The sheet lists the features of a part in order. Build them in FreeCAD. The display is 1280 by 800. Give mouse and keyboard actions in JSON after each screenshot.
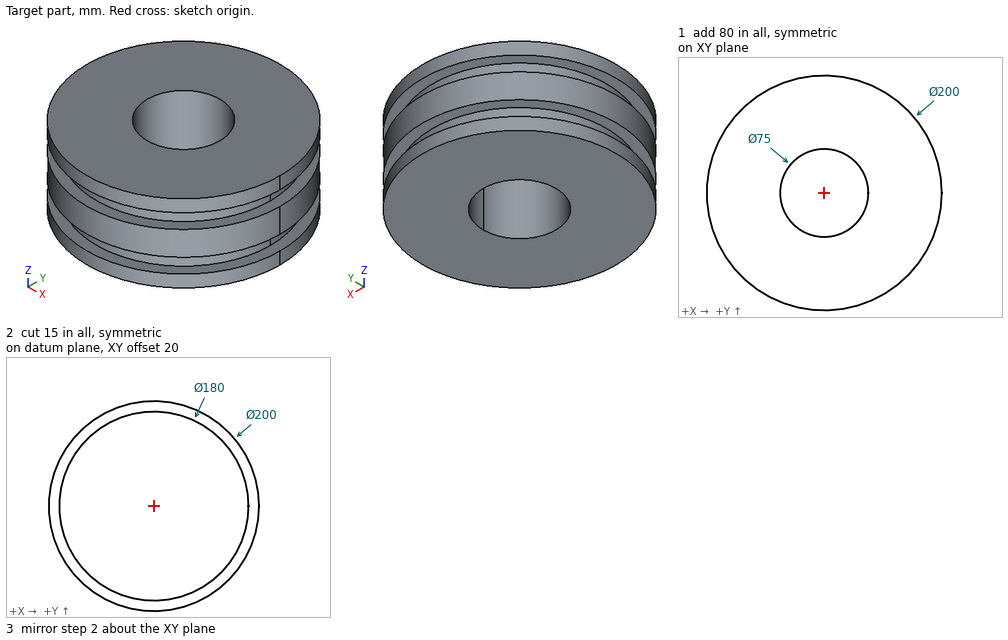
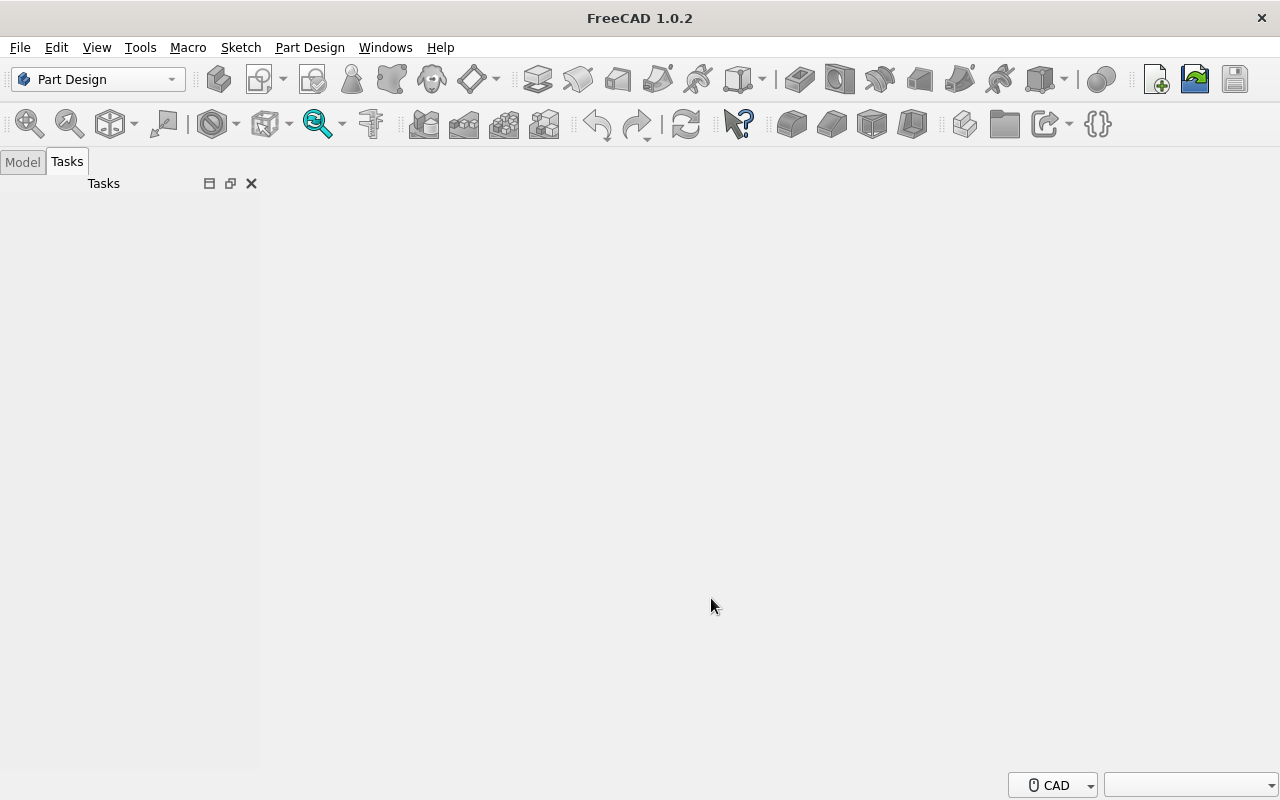
{"action": "left_click", "coordinate": [1156, 80]}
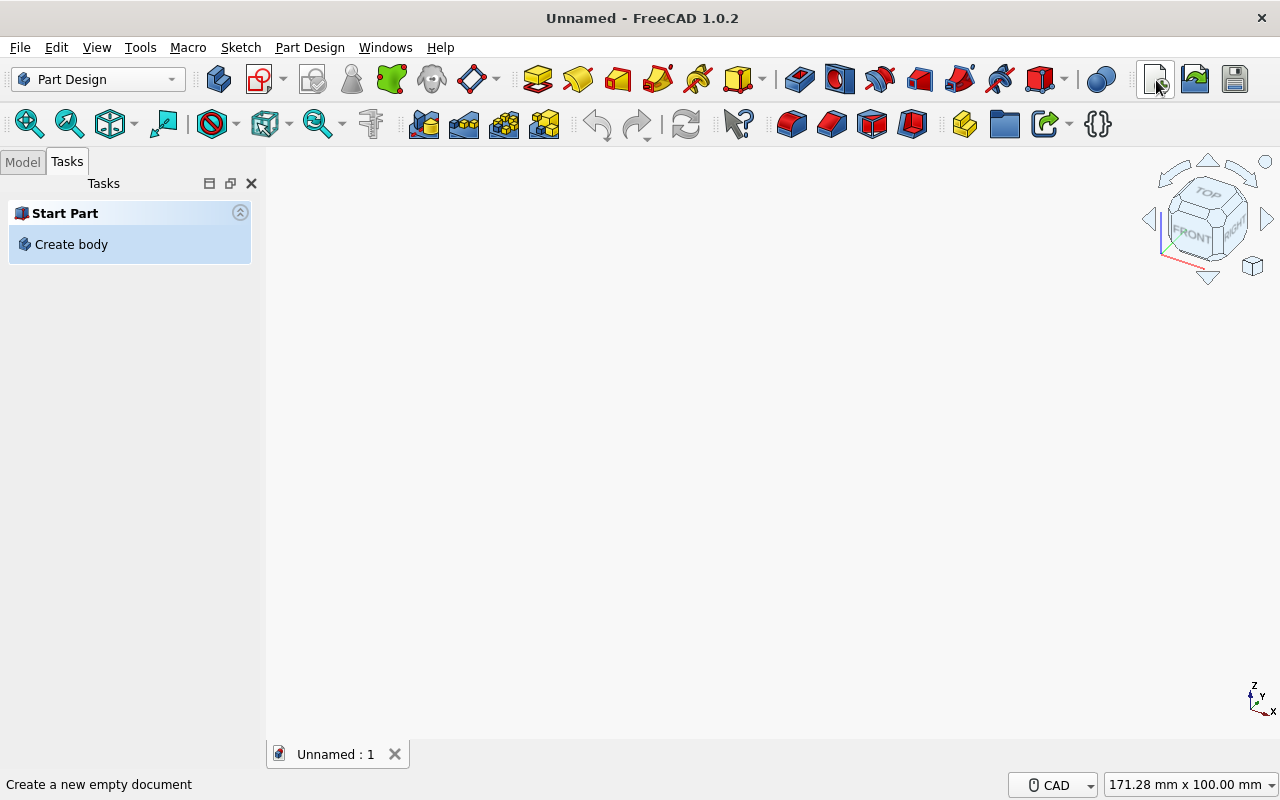
{"action": "left_click", "coordinate": [260, 80]}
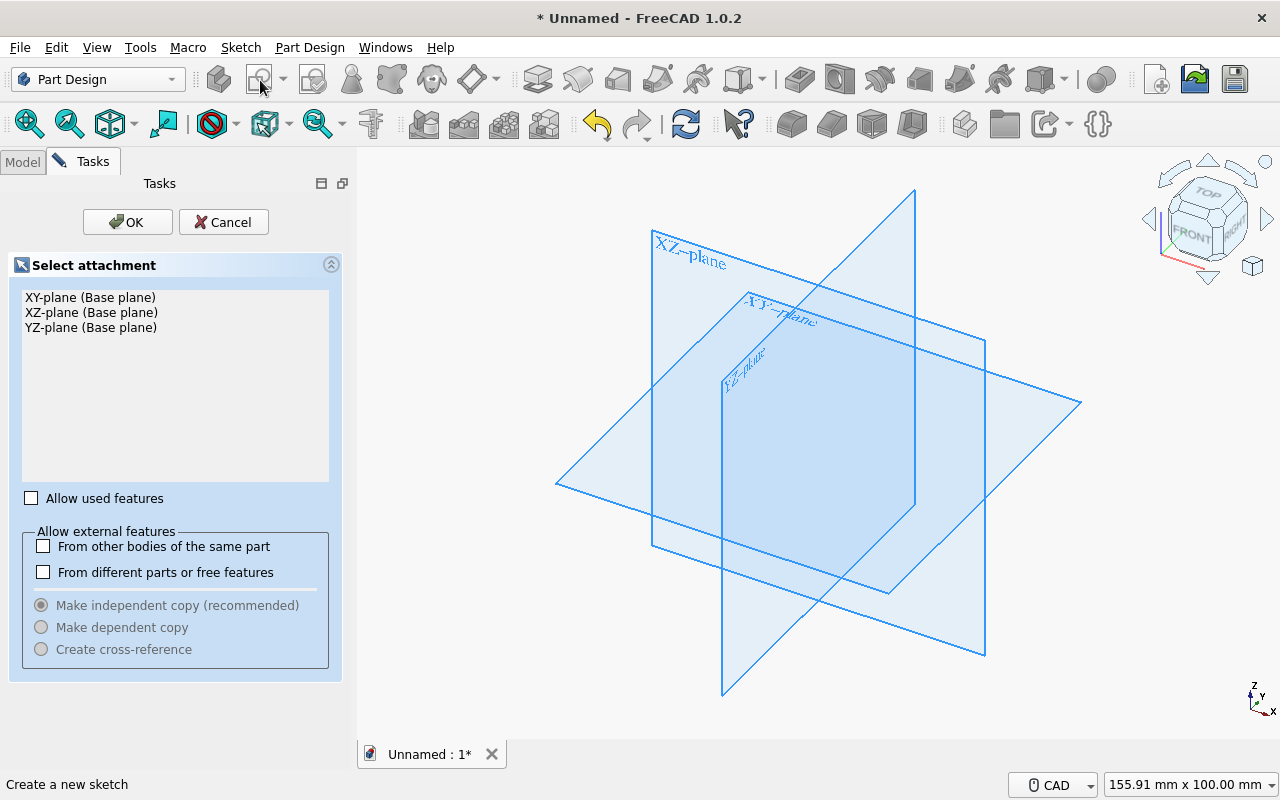
{"action": "left_click", "coordinate": [82, 298]}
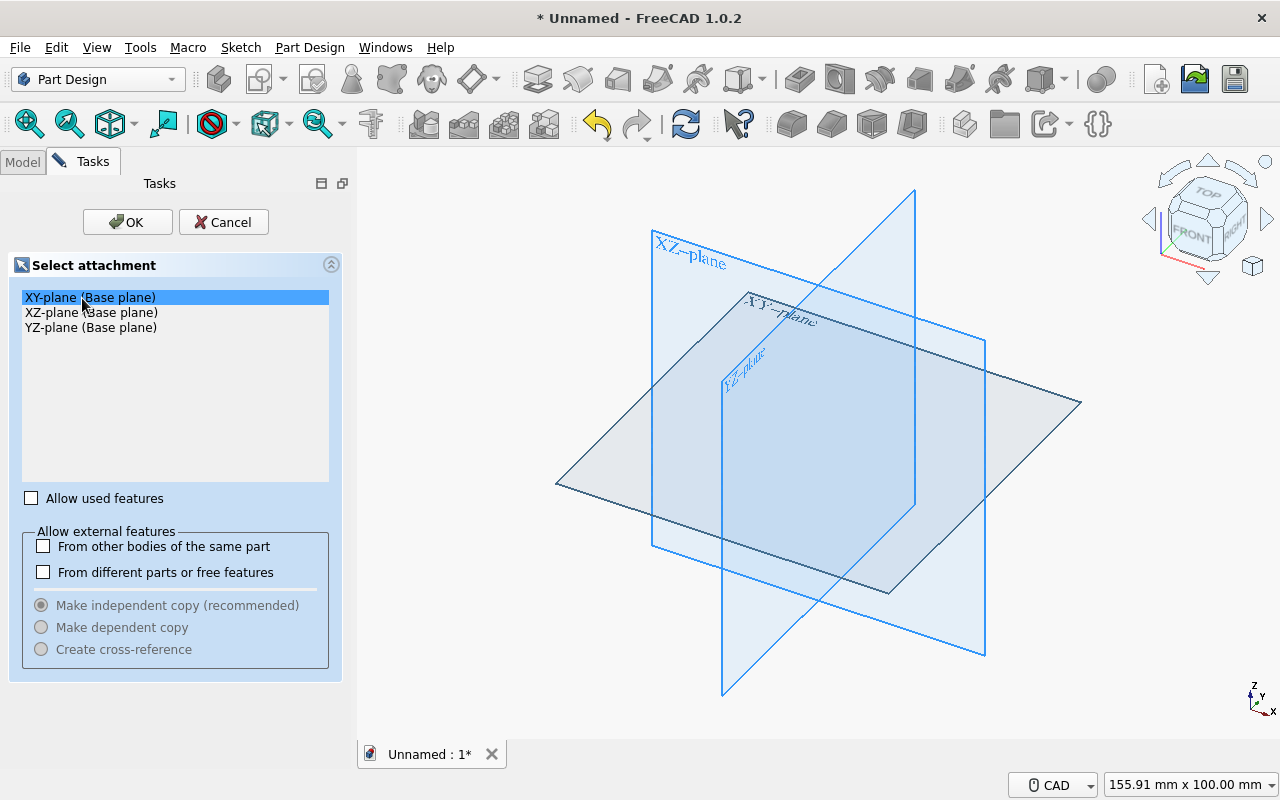
{"action": "left_click", "coordinate": [128, 222]}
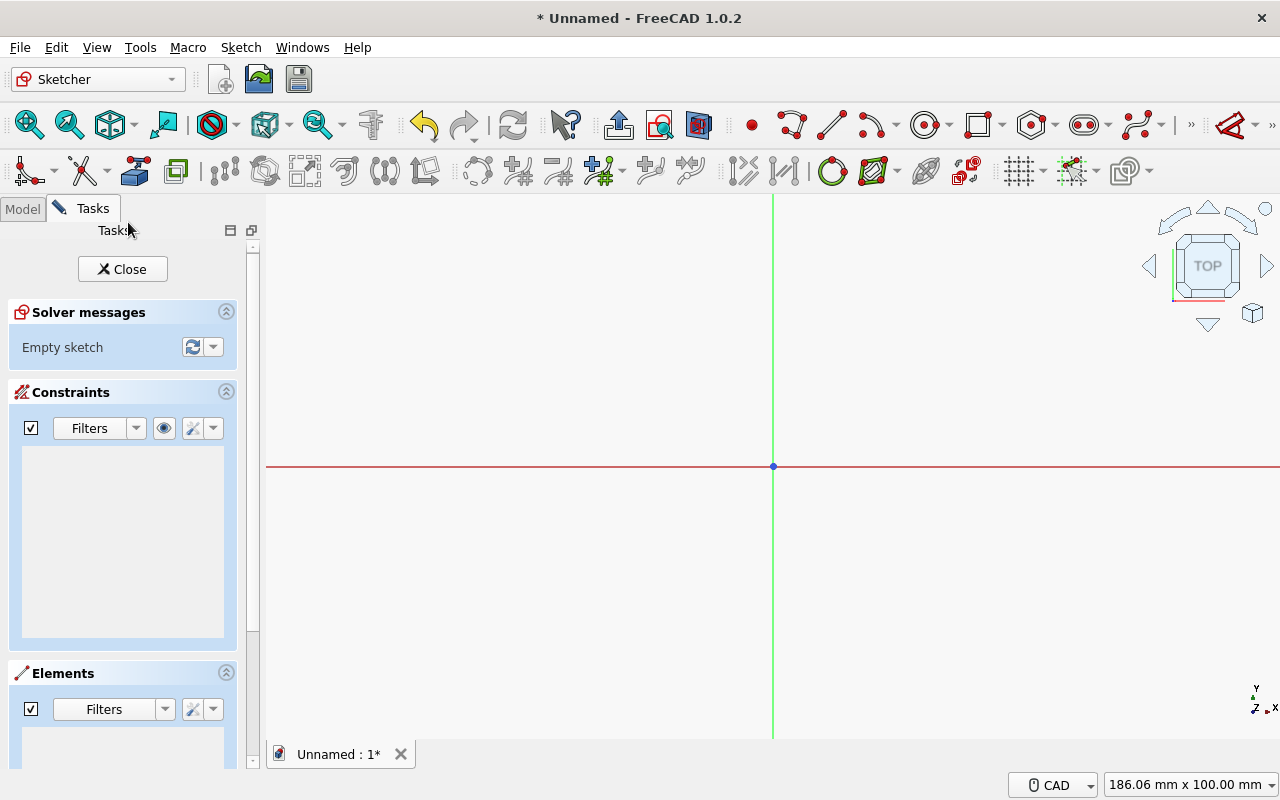
{"action": "scroll", "coordinate": [675, 466], "scroll_direction": "down", "scroll_amount": 6}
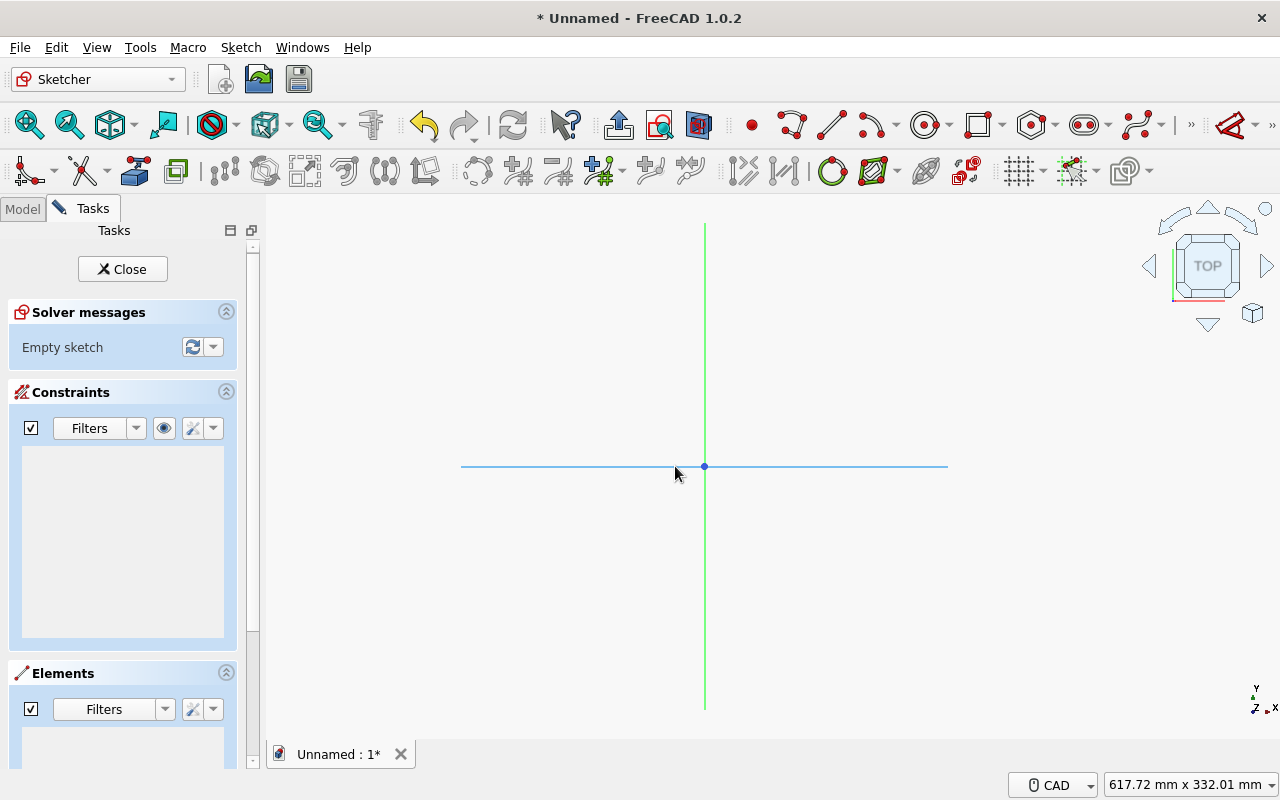
{"action": "left_click", "coordinate": [926, 126]}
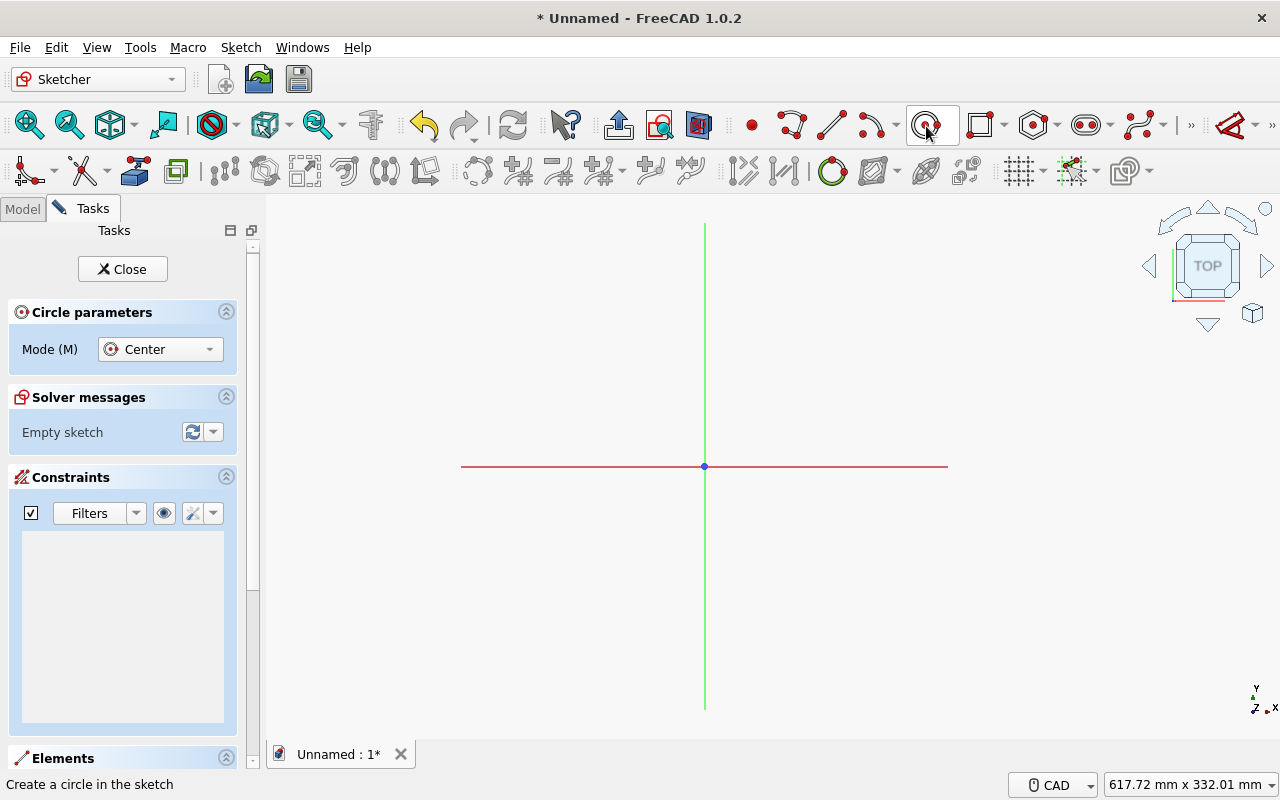
{"action": "left_click", "coordinate": [705, 466]}
{"action": "left_click", "coordinate": [821, 350]}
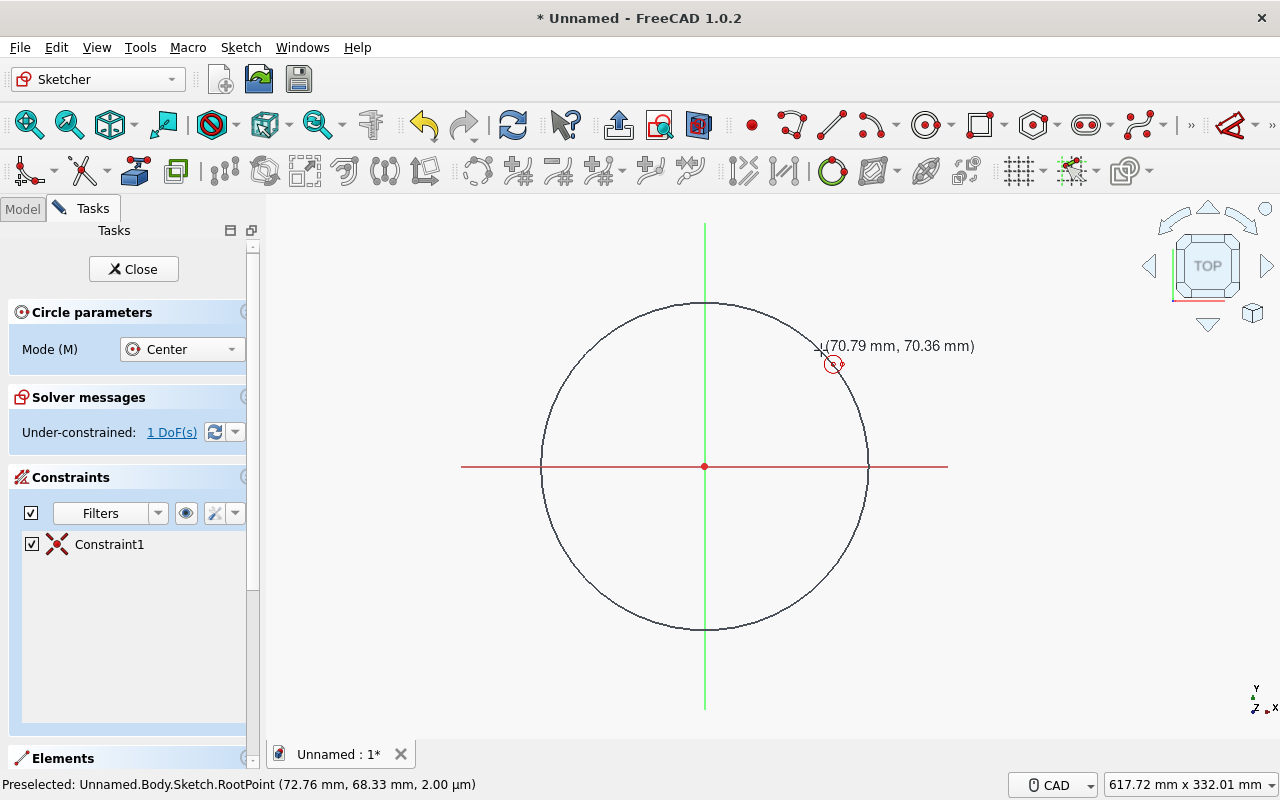
{"action": "left_click", "coordinate": [705, 466]}
{"action": "left_click", "coordinate": [748, 423]}
{"action": "key", "text": "Escape"}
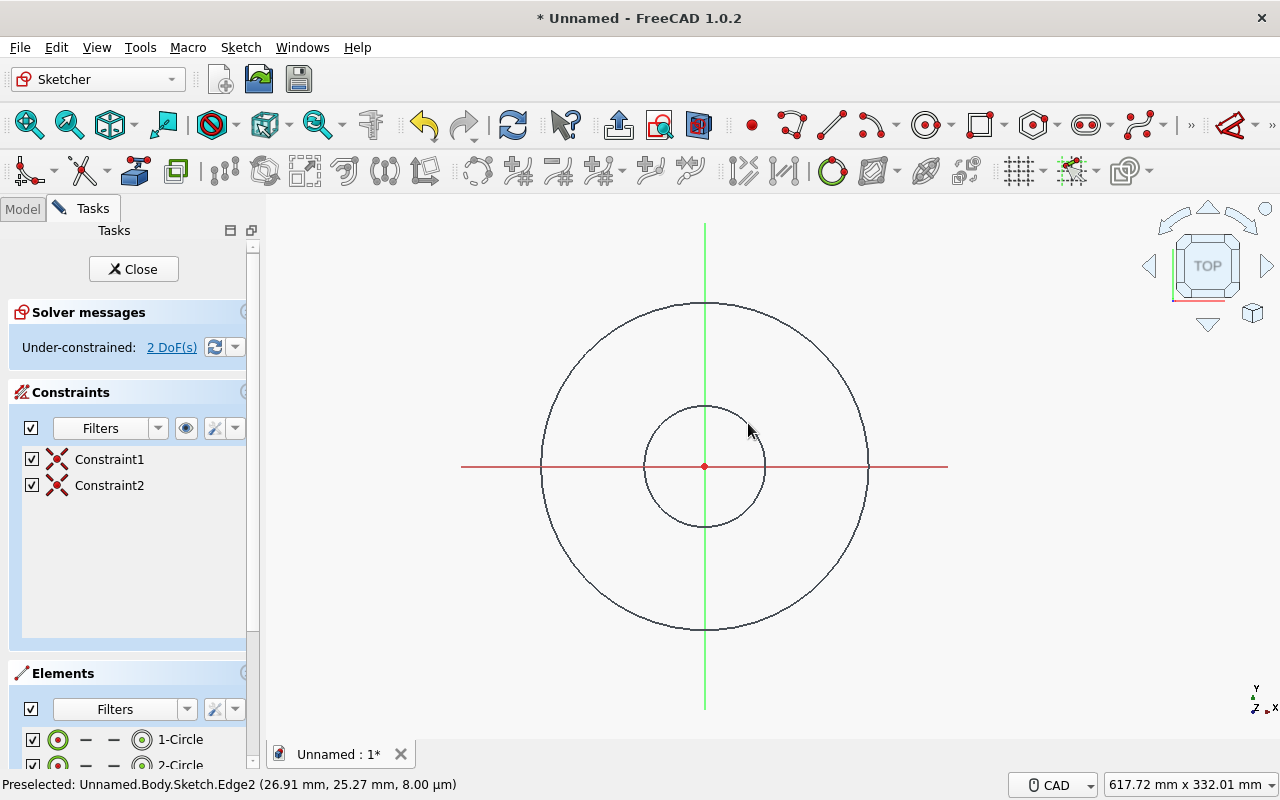
{"action": "left_click", "coordinate": [1230, 126]}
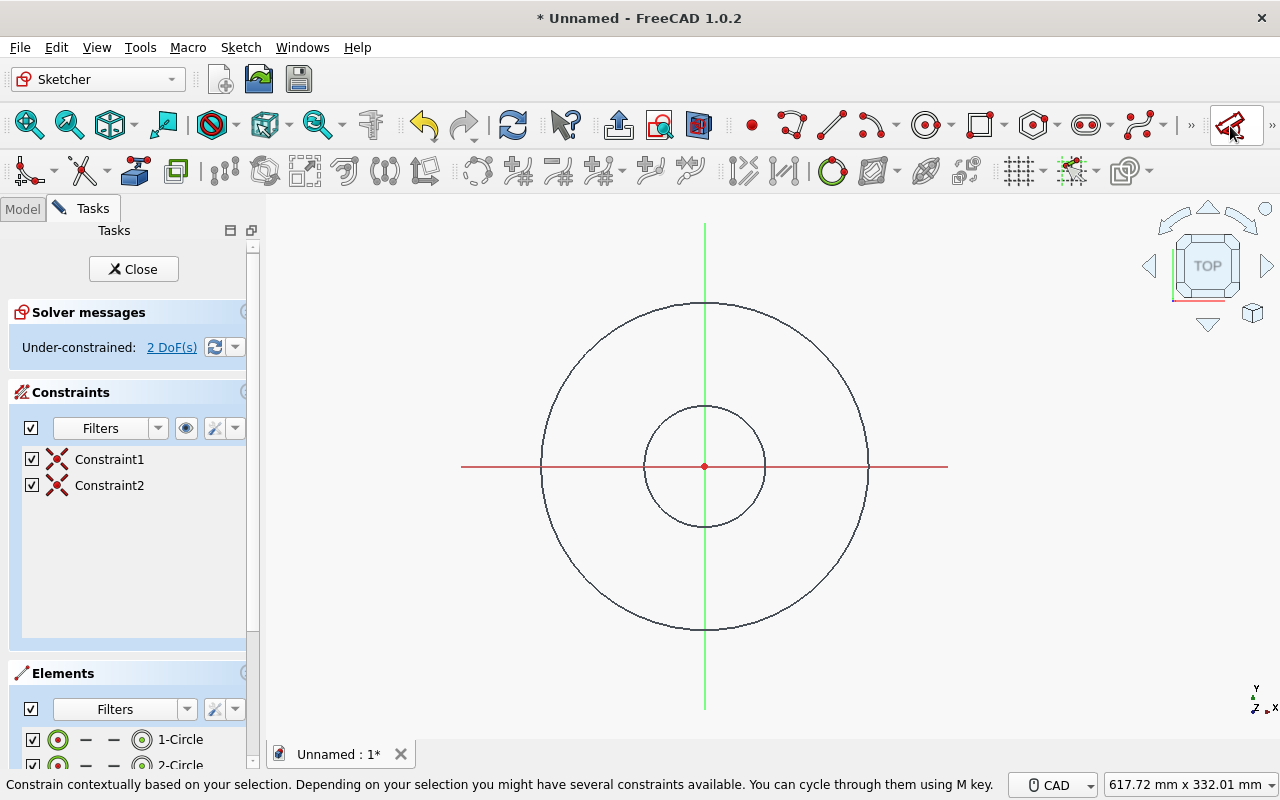
{"action": "left_click", "coordinate": [820, 350]}
{"action": "left_click", "coordinate": [843, 327]}